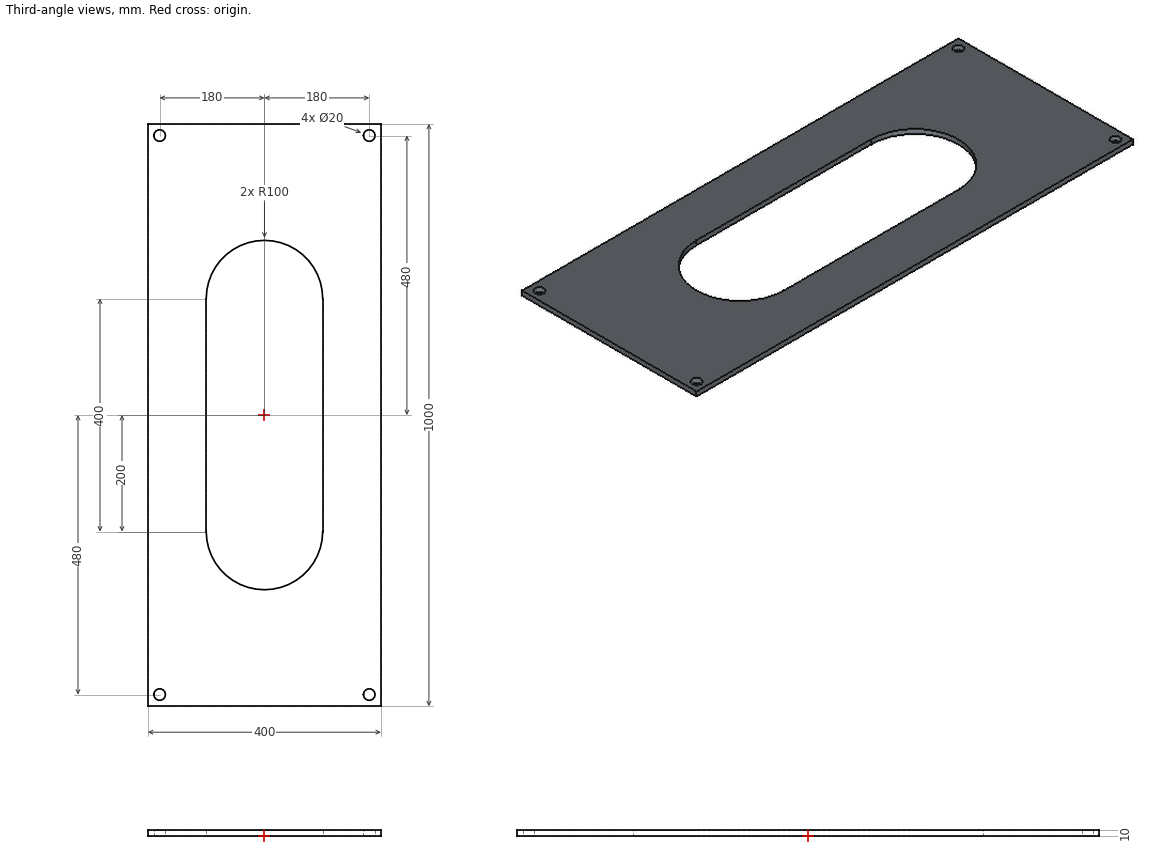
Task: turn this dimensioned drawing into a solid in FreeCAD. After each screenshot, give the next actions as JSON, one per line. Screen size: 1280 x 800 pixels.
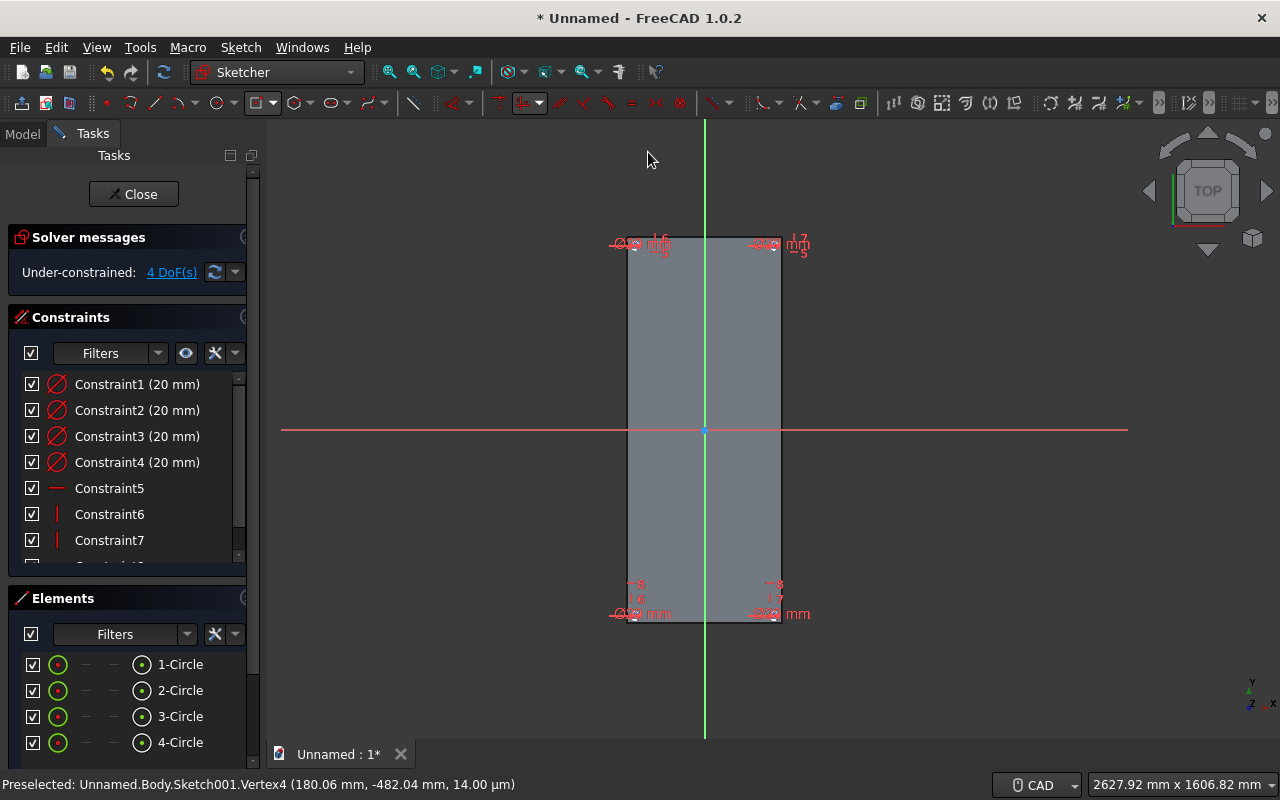
{"action": "left_click", "coordinate": [774, 246]}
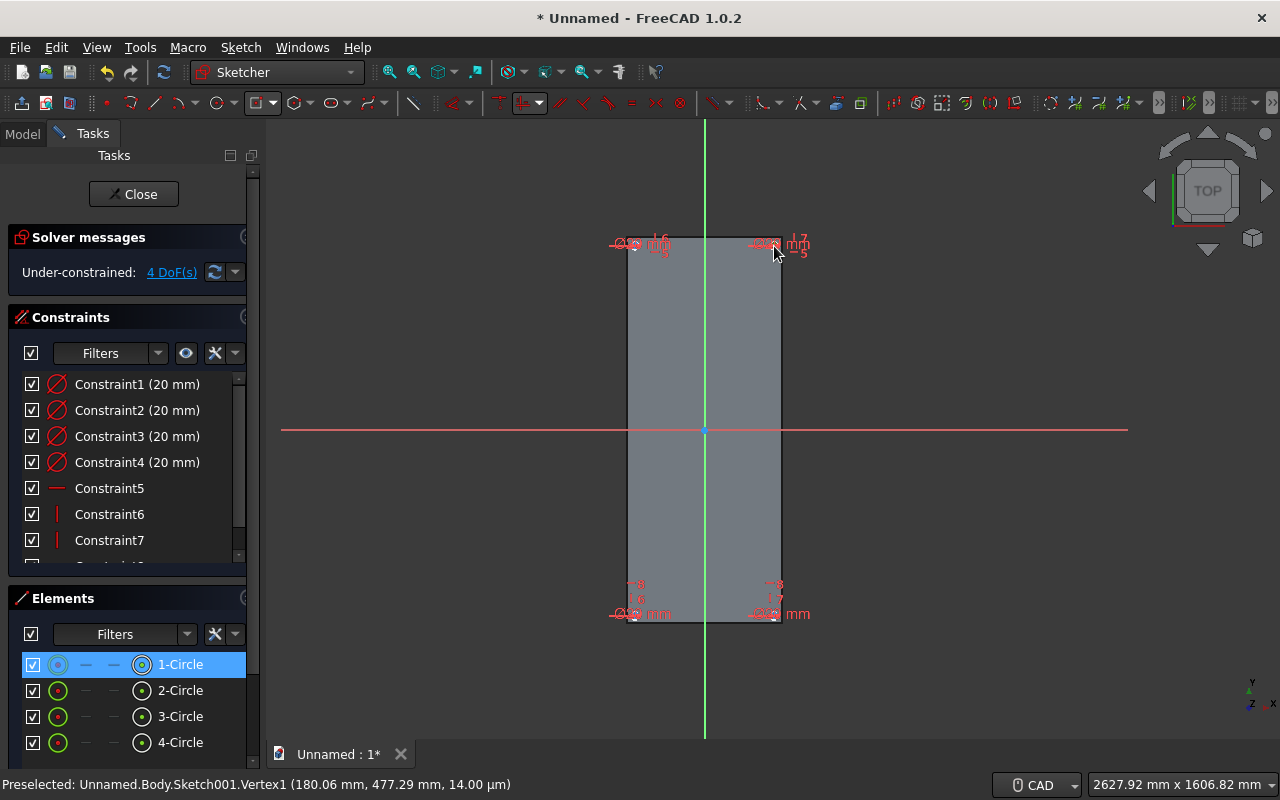
{"action": "left_click", "coordinate": [472, 104]}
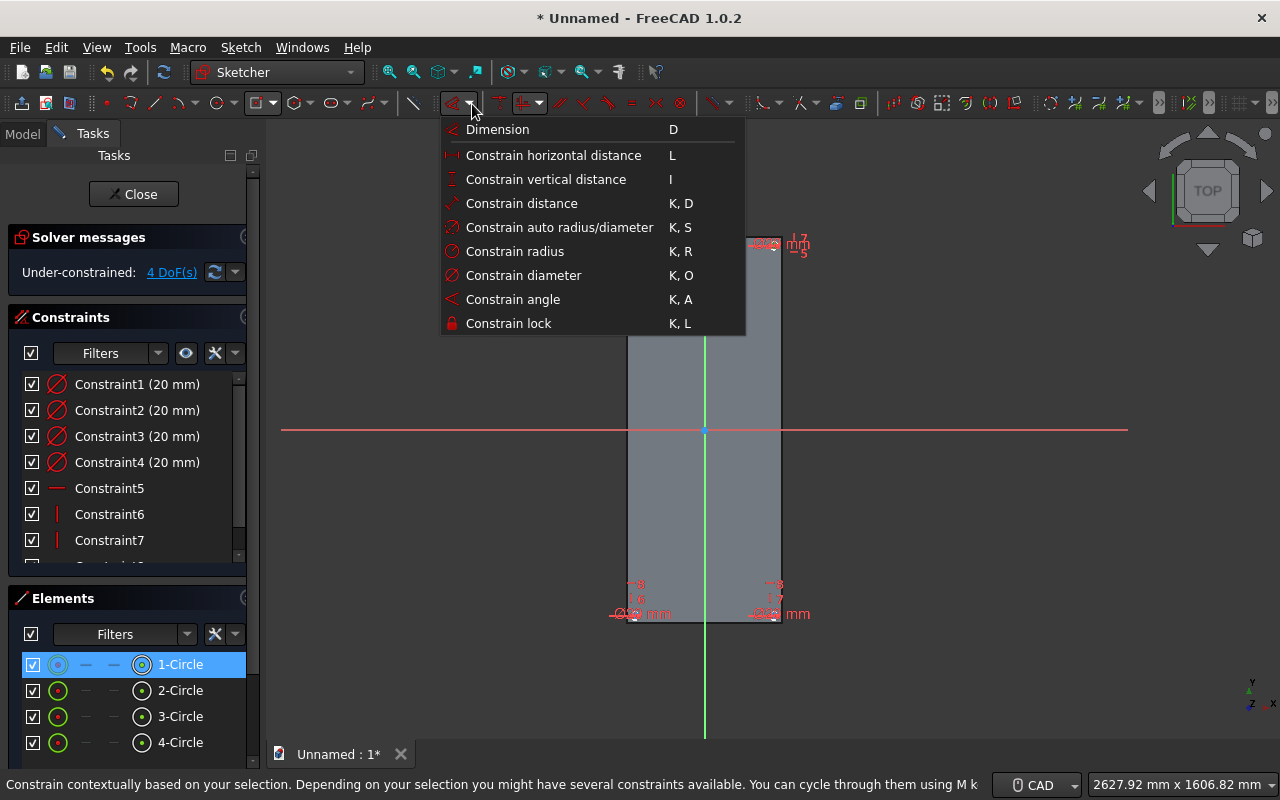
{"action": "left_click", "coordinate": [593, 155]}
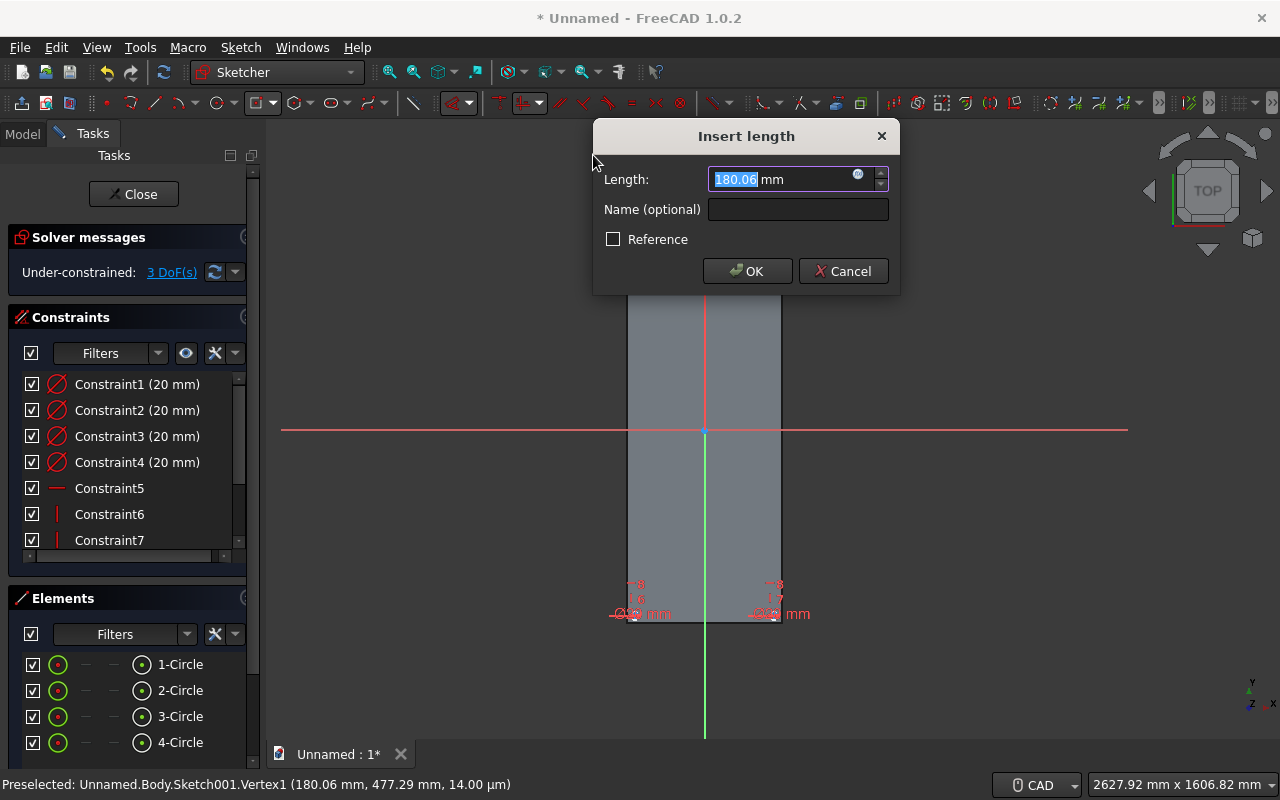
{"action": "type", "text": "180"}
{"action": "key", "text": "Return"}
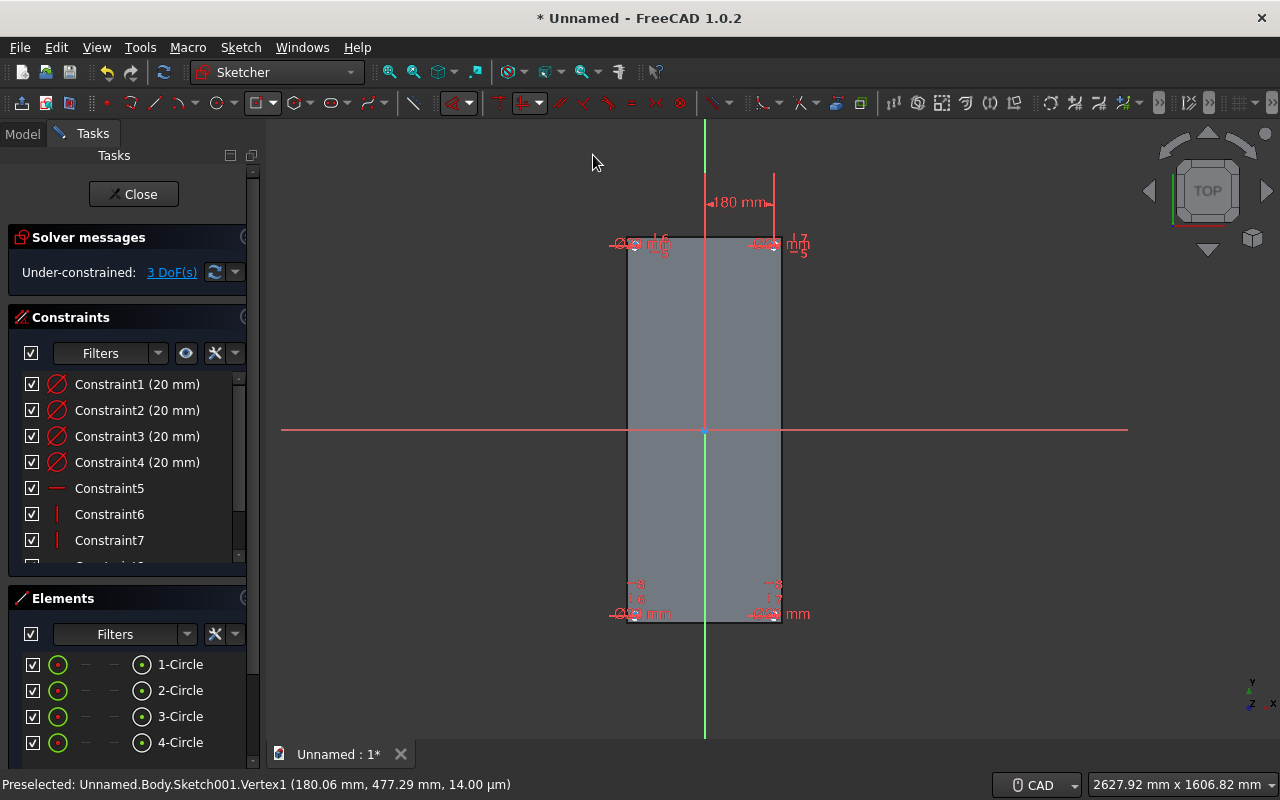
{"action": "left_click", "coordinate": [774, 246]}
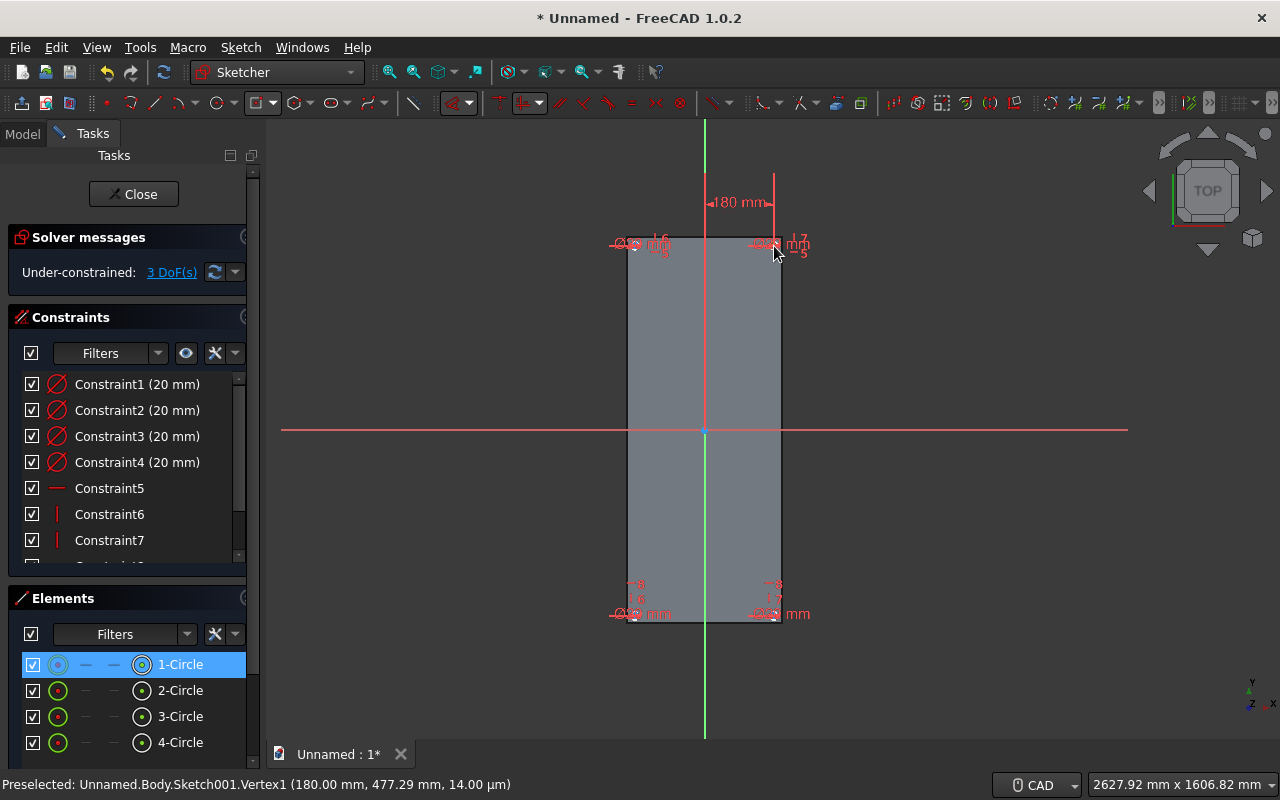
{"action": "left_click", "coordinate": [472, 104]}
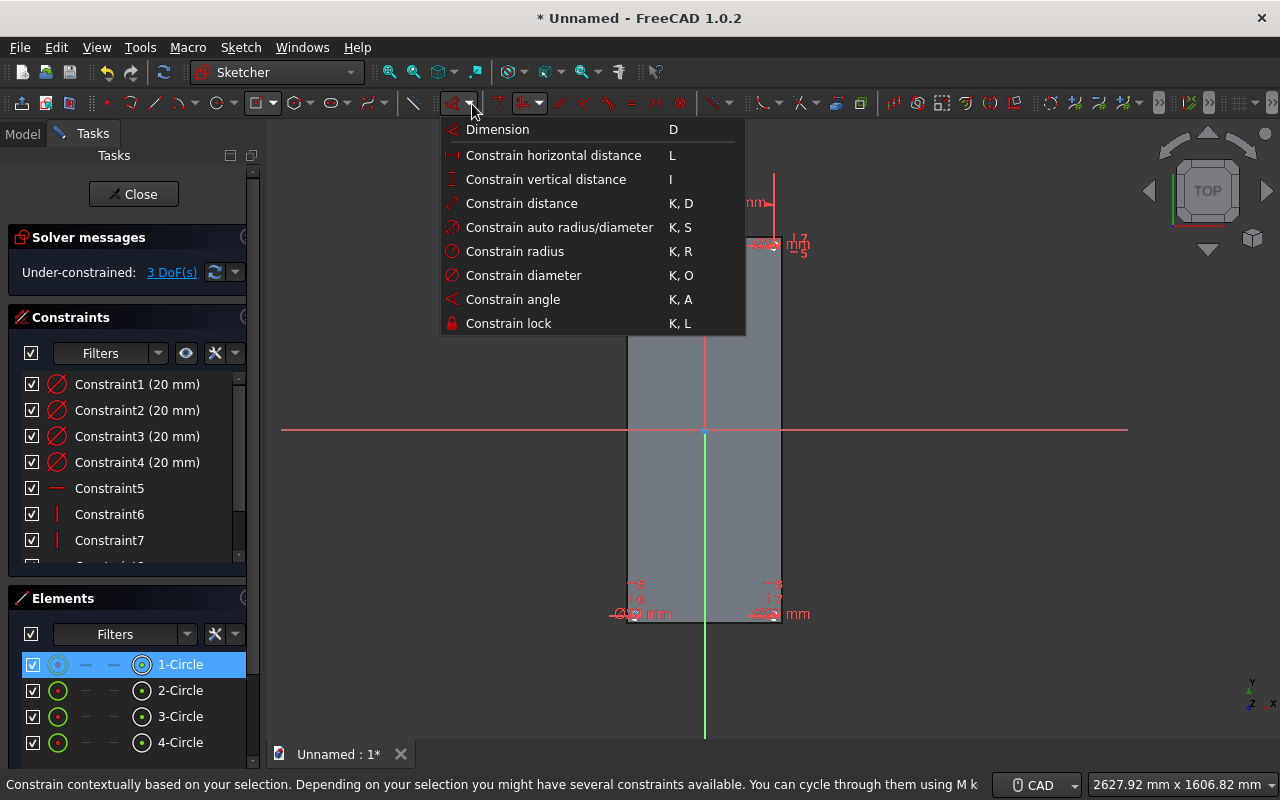
{"action": "left_click", "coordinate": [593, 179]}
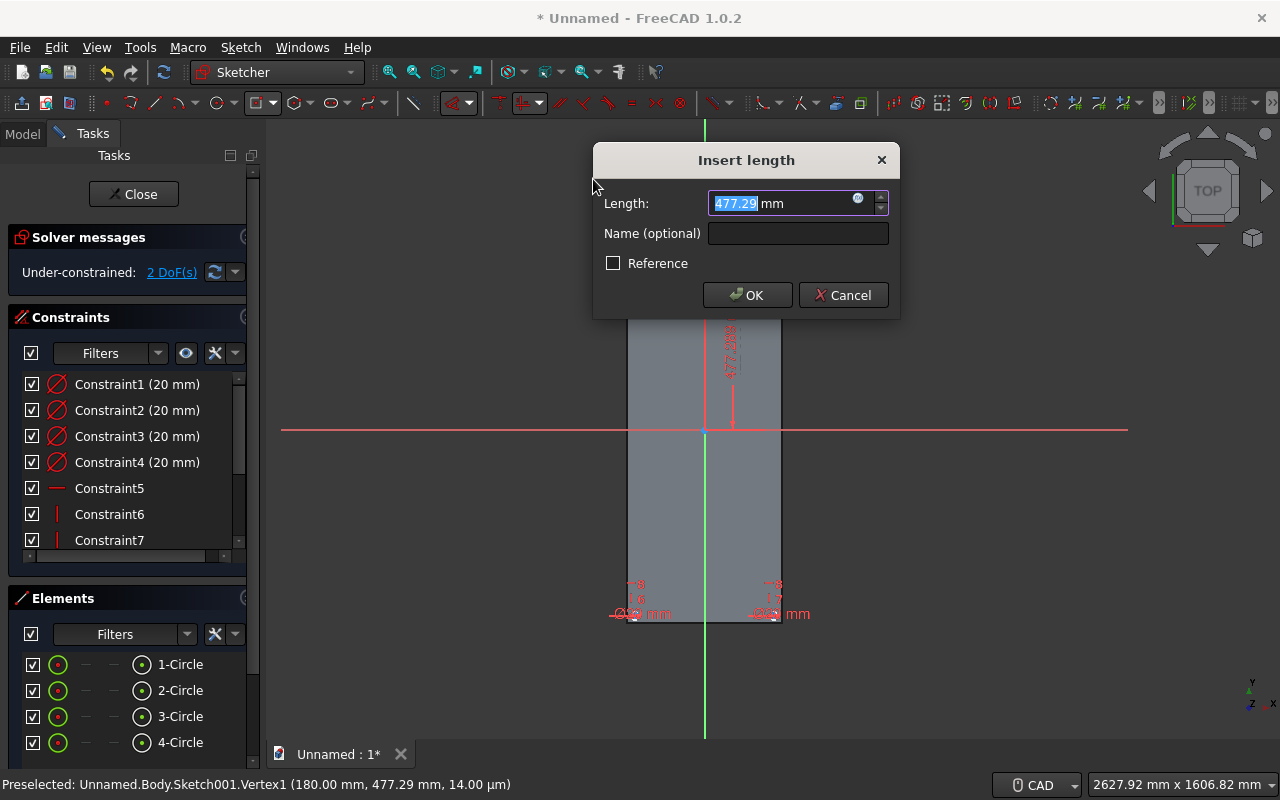
{"action": "type", "text": "480"}
{"action": "key", "text": "Return"}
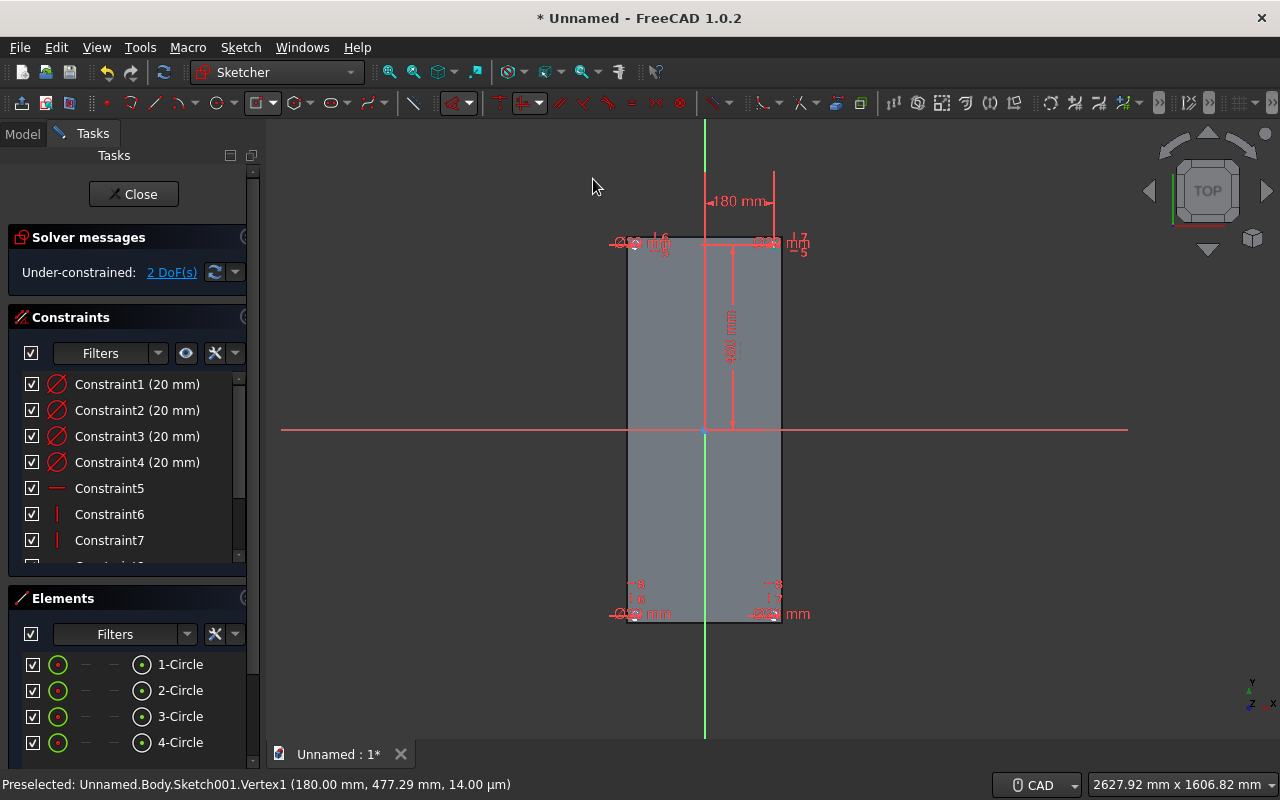
{"action": "left_click", "coordinate": [635, 245]}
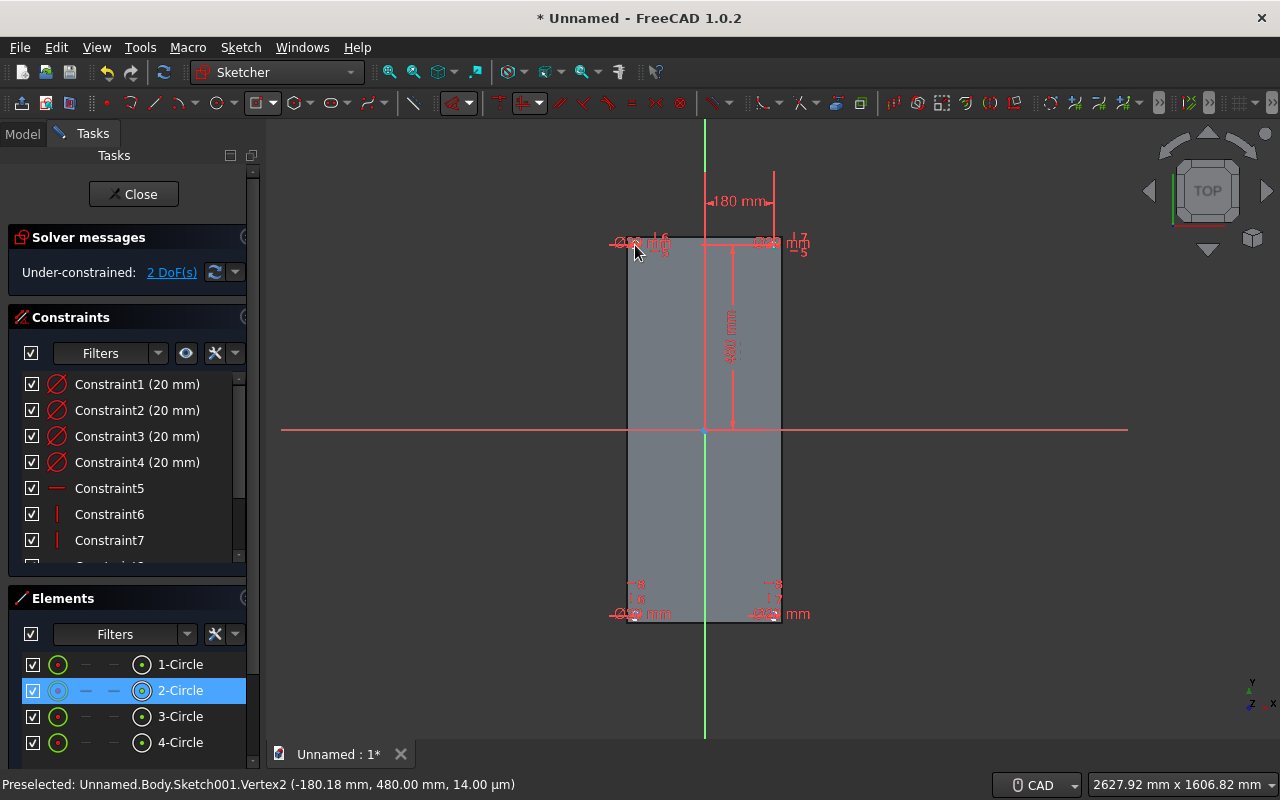
{"action": "left_click", "coordinate": [472, 104]}